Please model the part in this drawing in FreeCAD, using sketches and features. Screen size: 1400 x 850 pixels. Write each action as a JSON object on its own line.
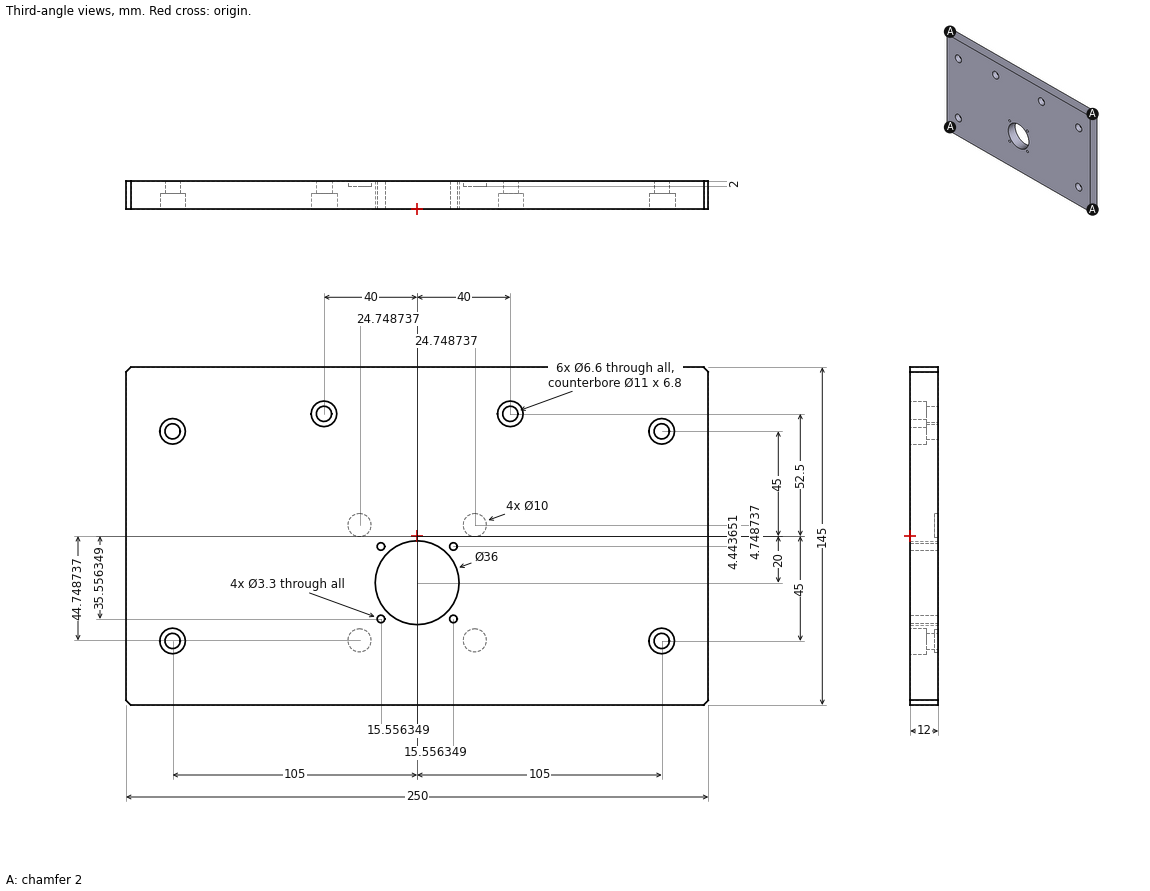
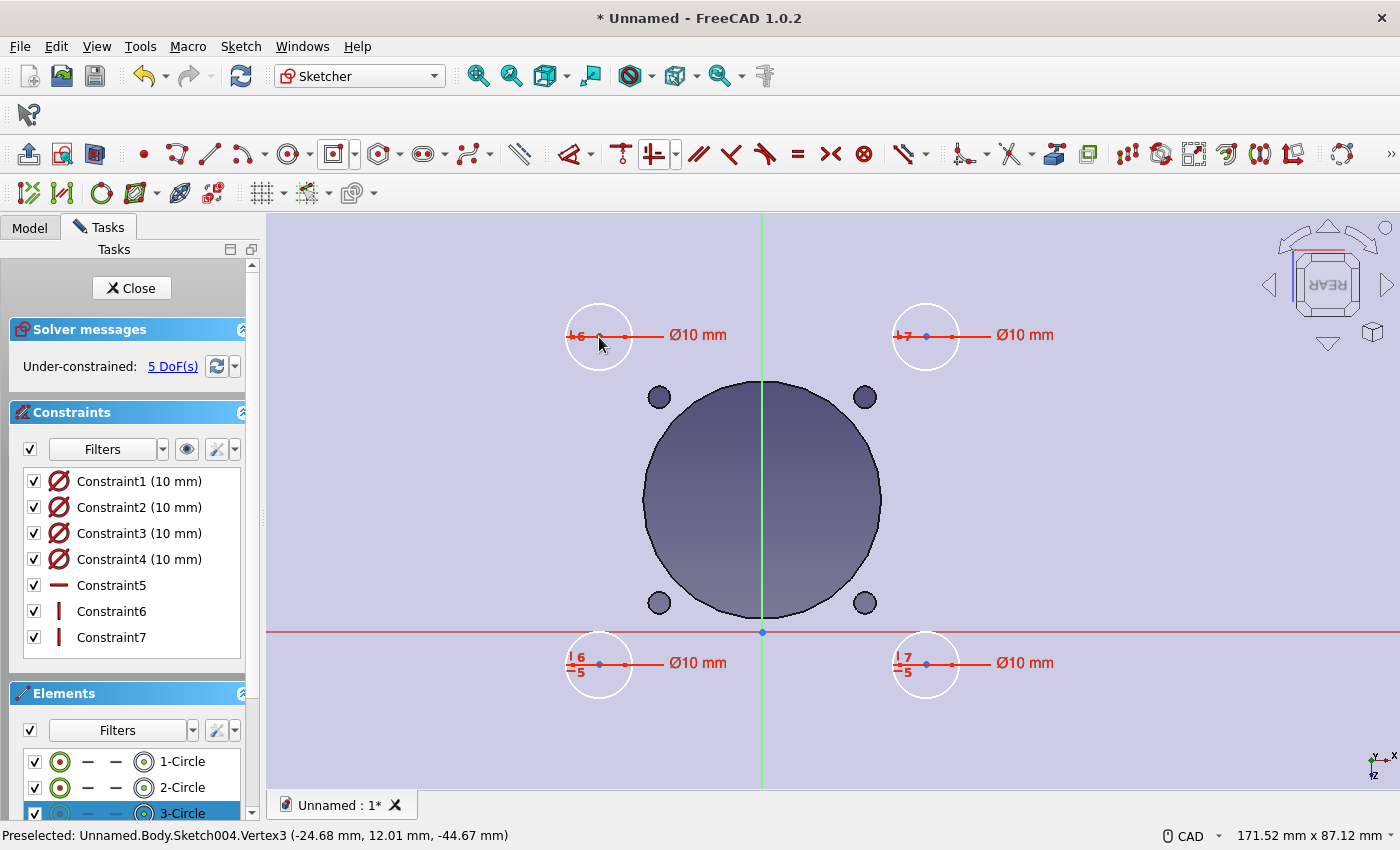
{"action": "left_click", "coordinate": [926, 337]}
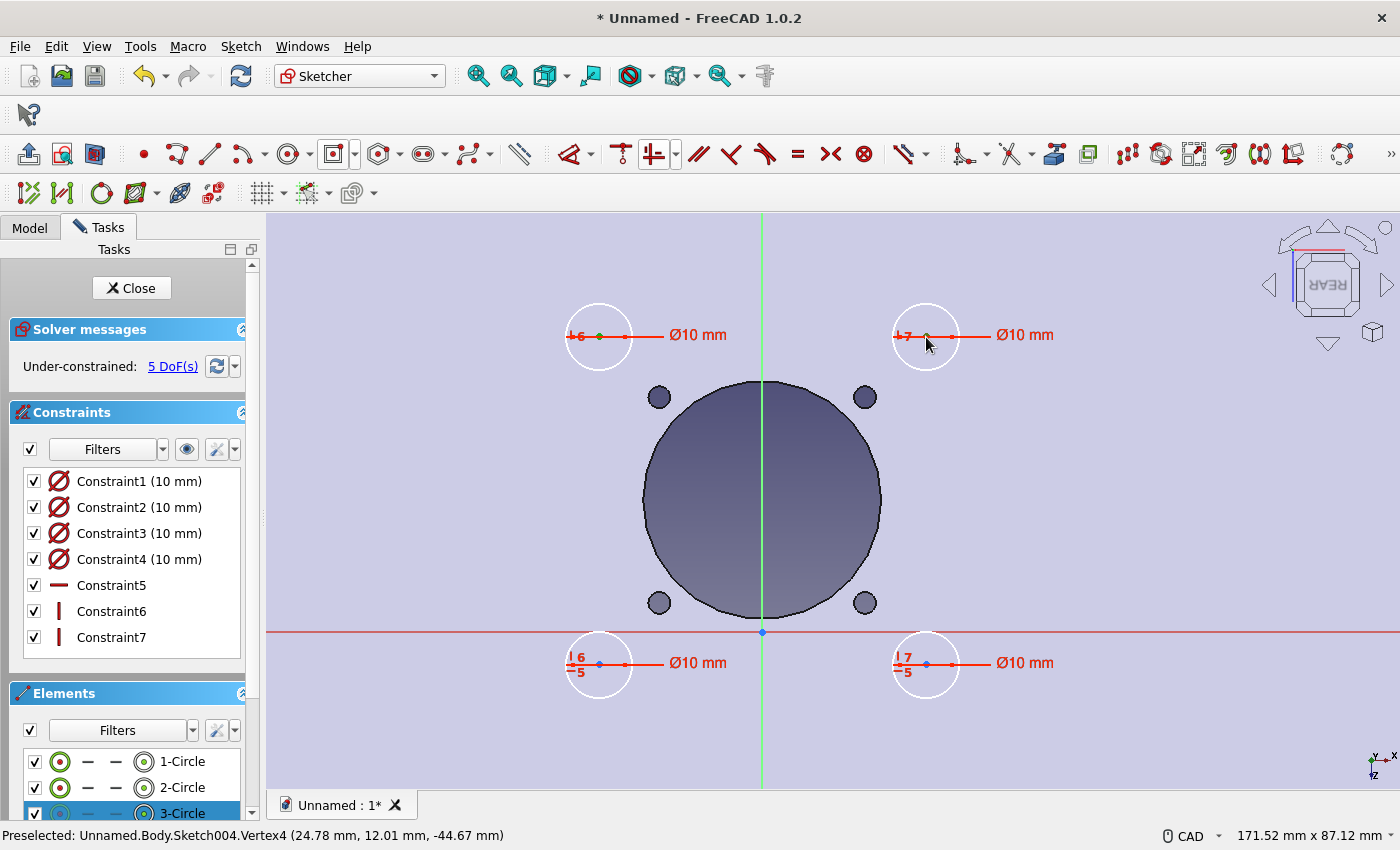
{"action": "key", "text": "h"}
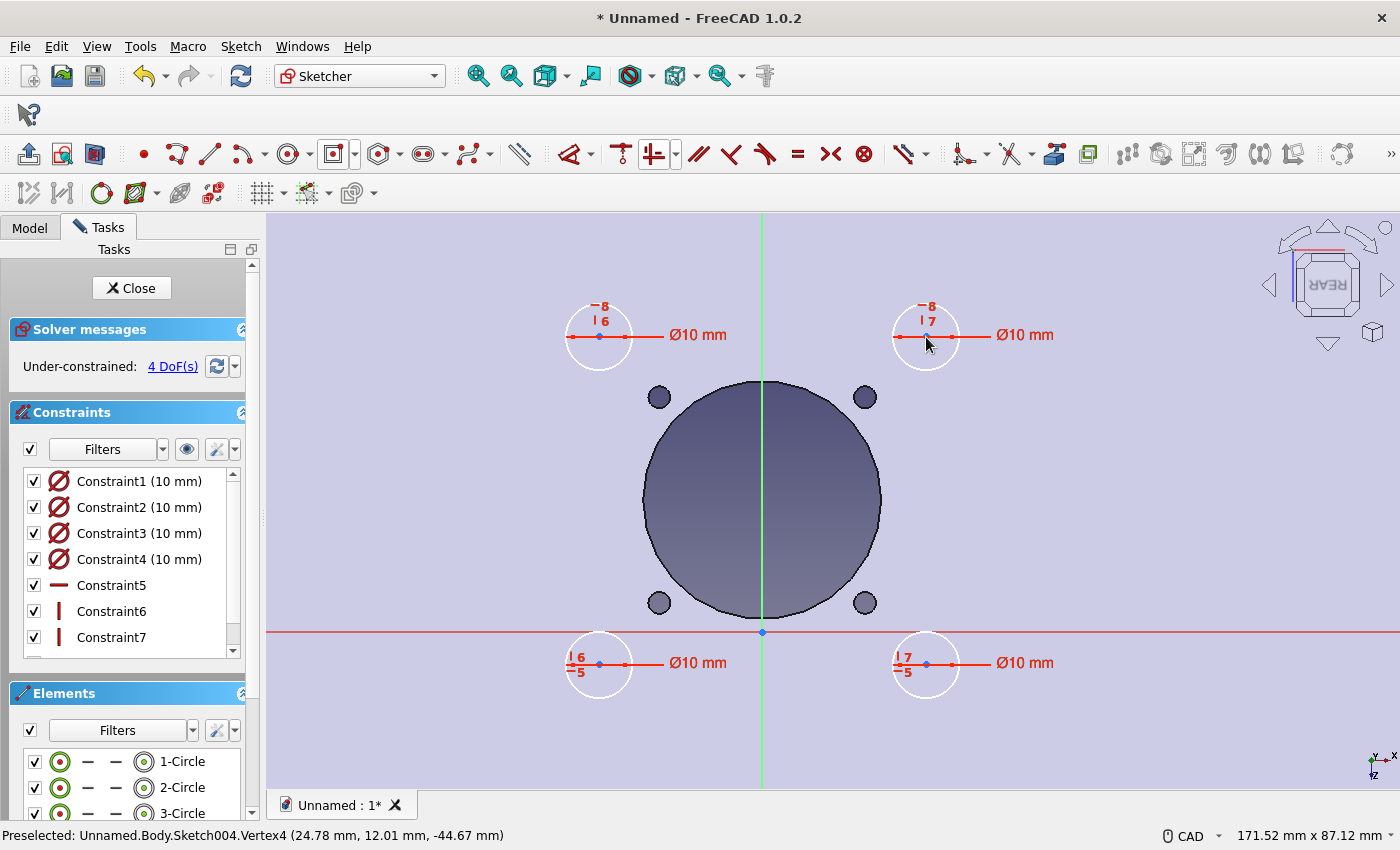
{"action": "left_click", "coordinate": [568, 154]}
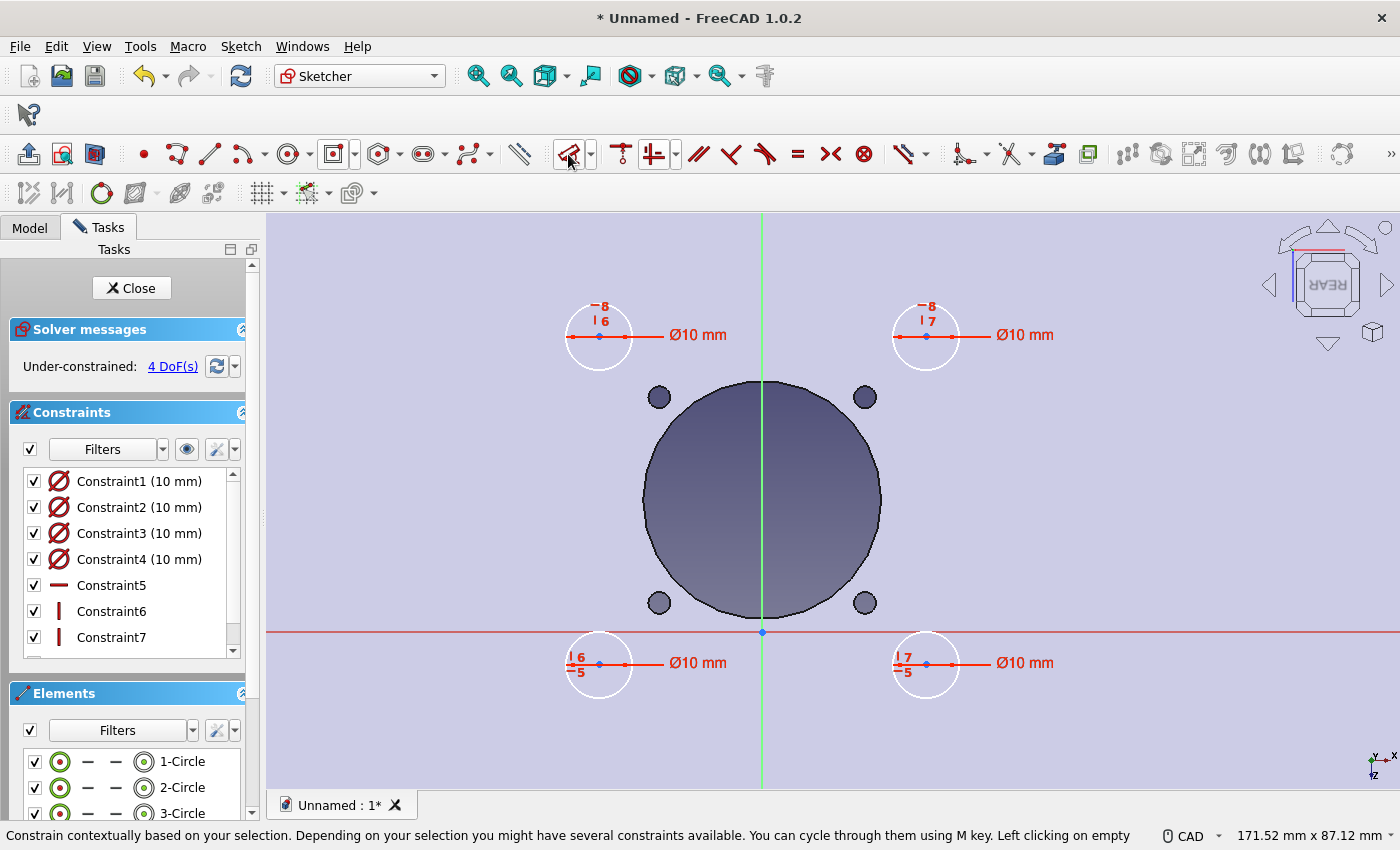
{"action": "scroll", "coordinate": [926, 665], "scroll_direction": "up", "scroll_amount": 2}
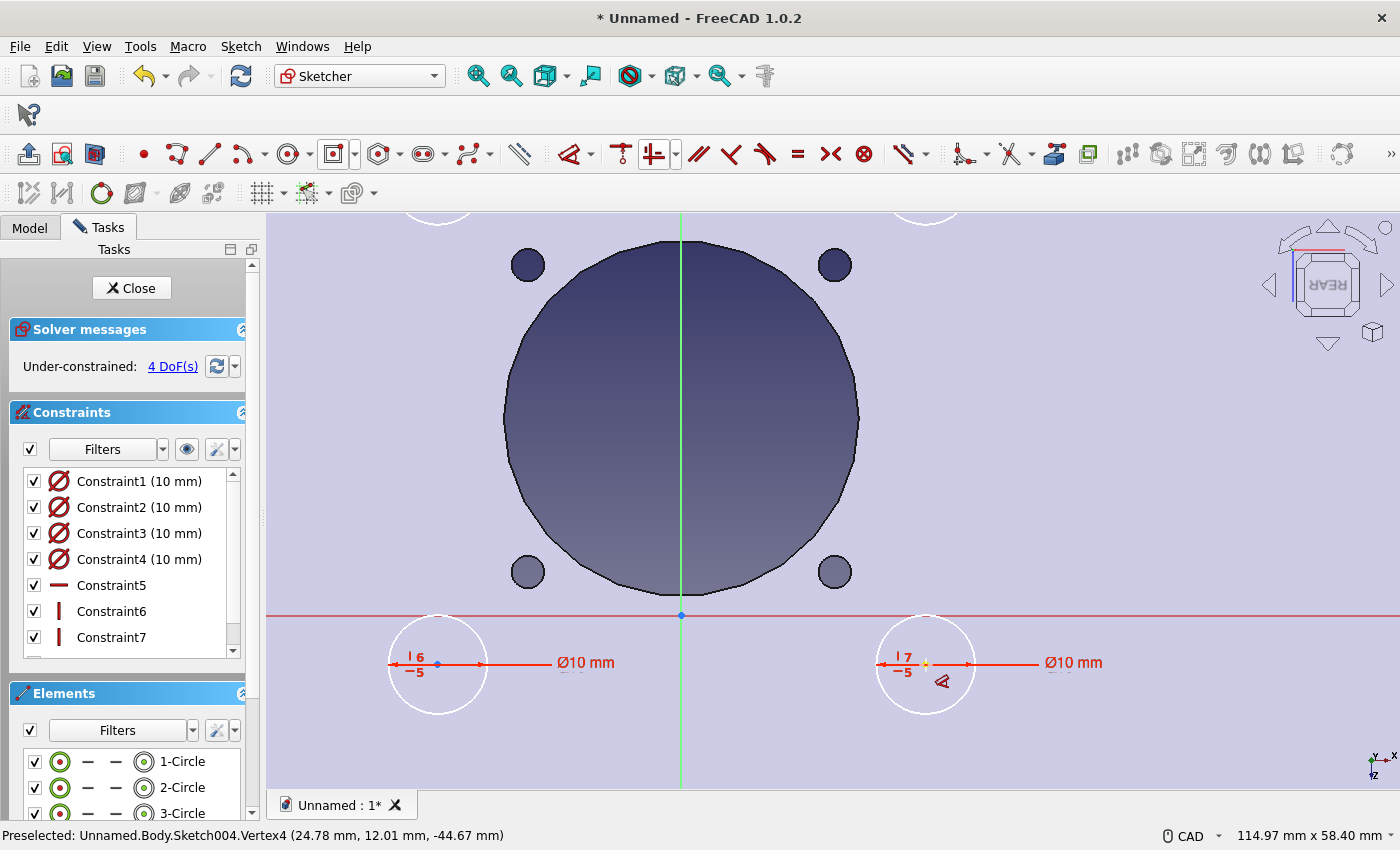
{"action": "left_click", "coordinate": [926, 665]}
{"action": "left_click", "coordinate": [960, 657]}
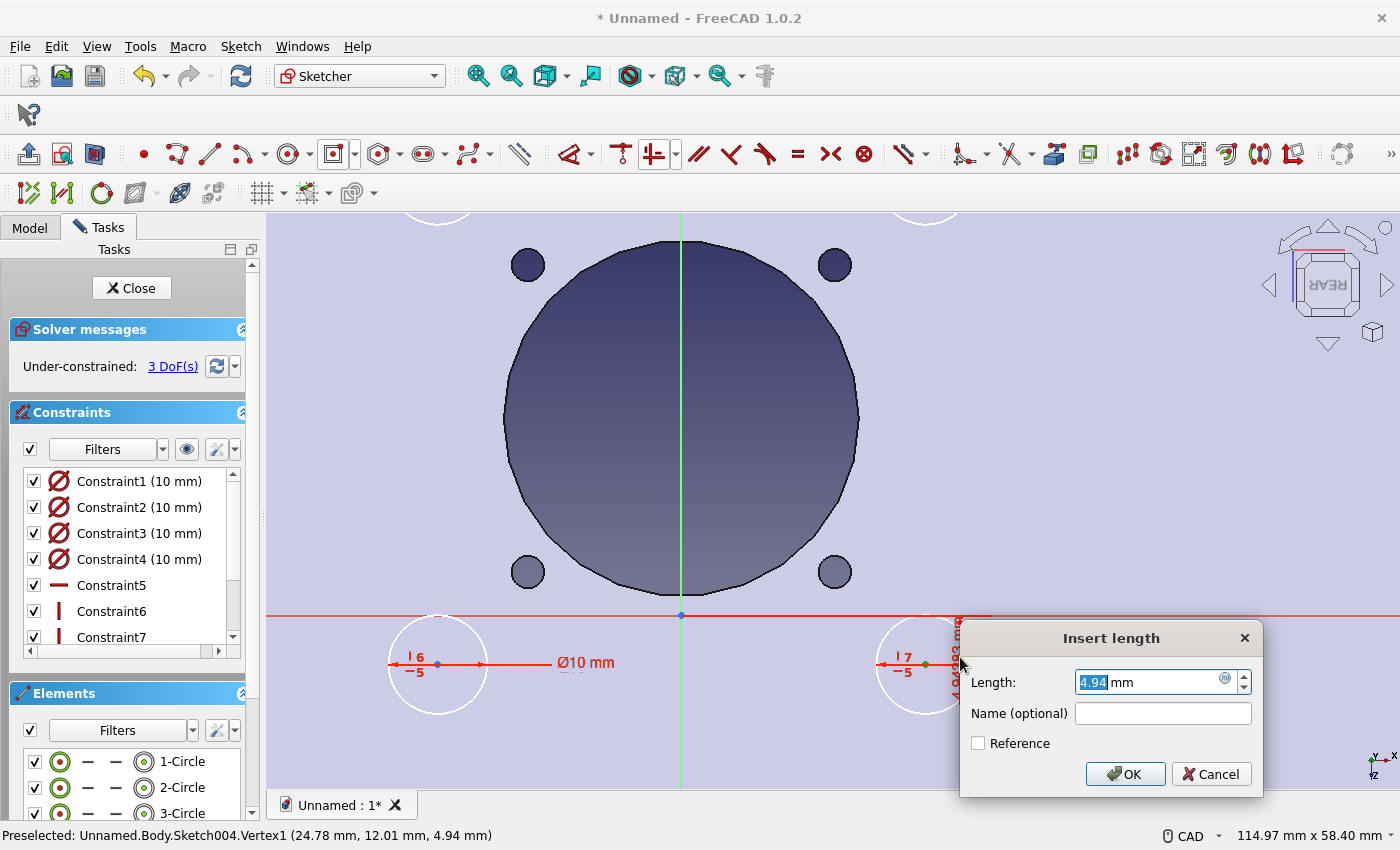
{"action": "type", "text": "4.748737"}
{"action": "key", "text": "Return"}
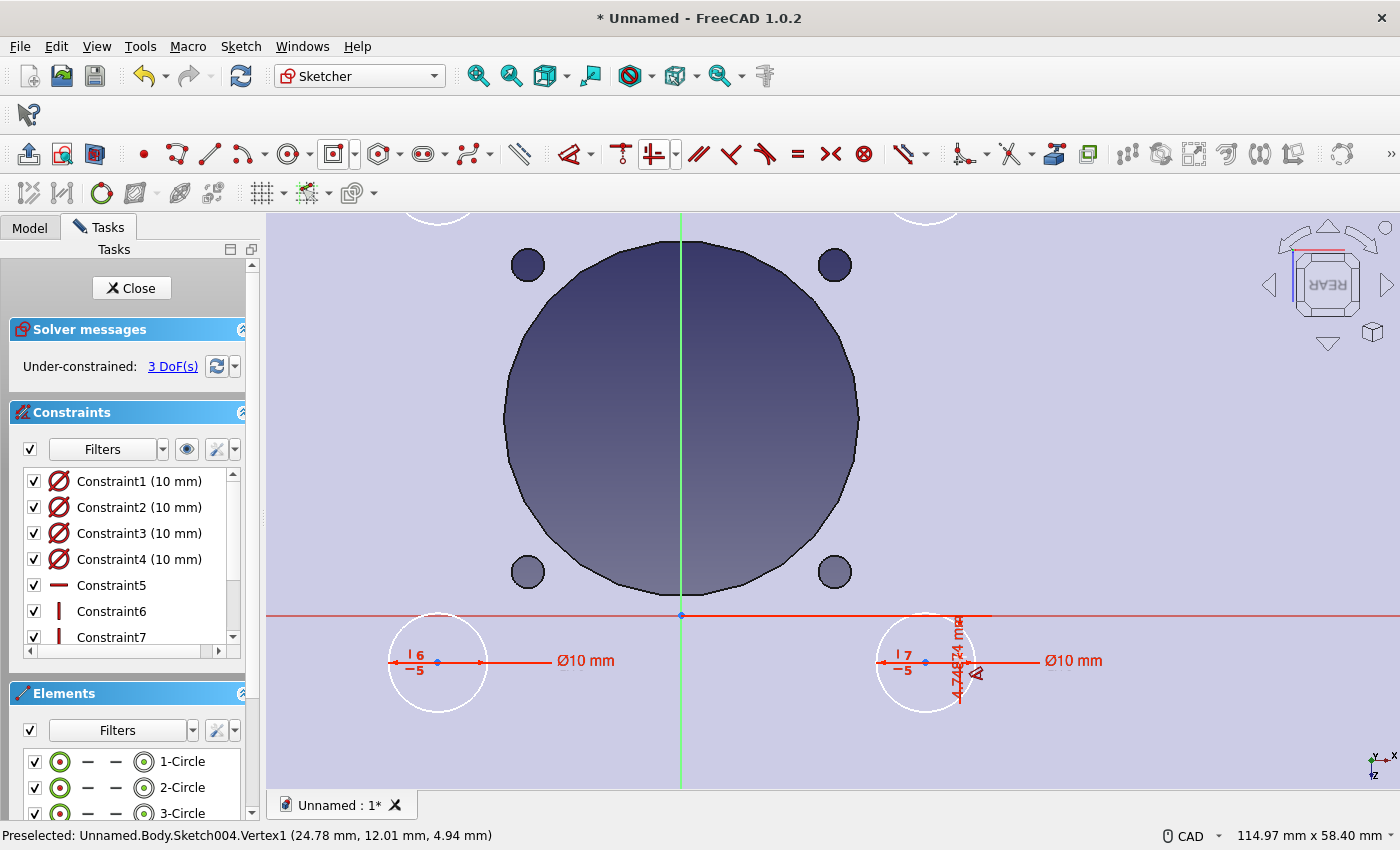
{"action": "left_click", "coordinate": [926, 663]}
{"action": "left_click", "coordinate": [804, 697]}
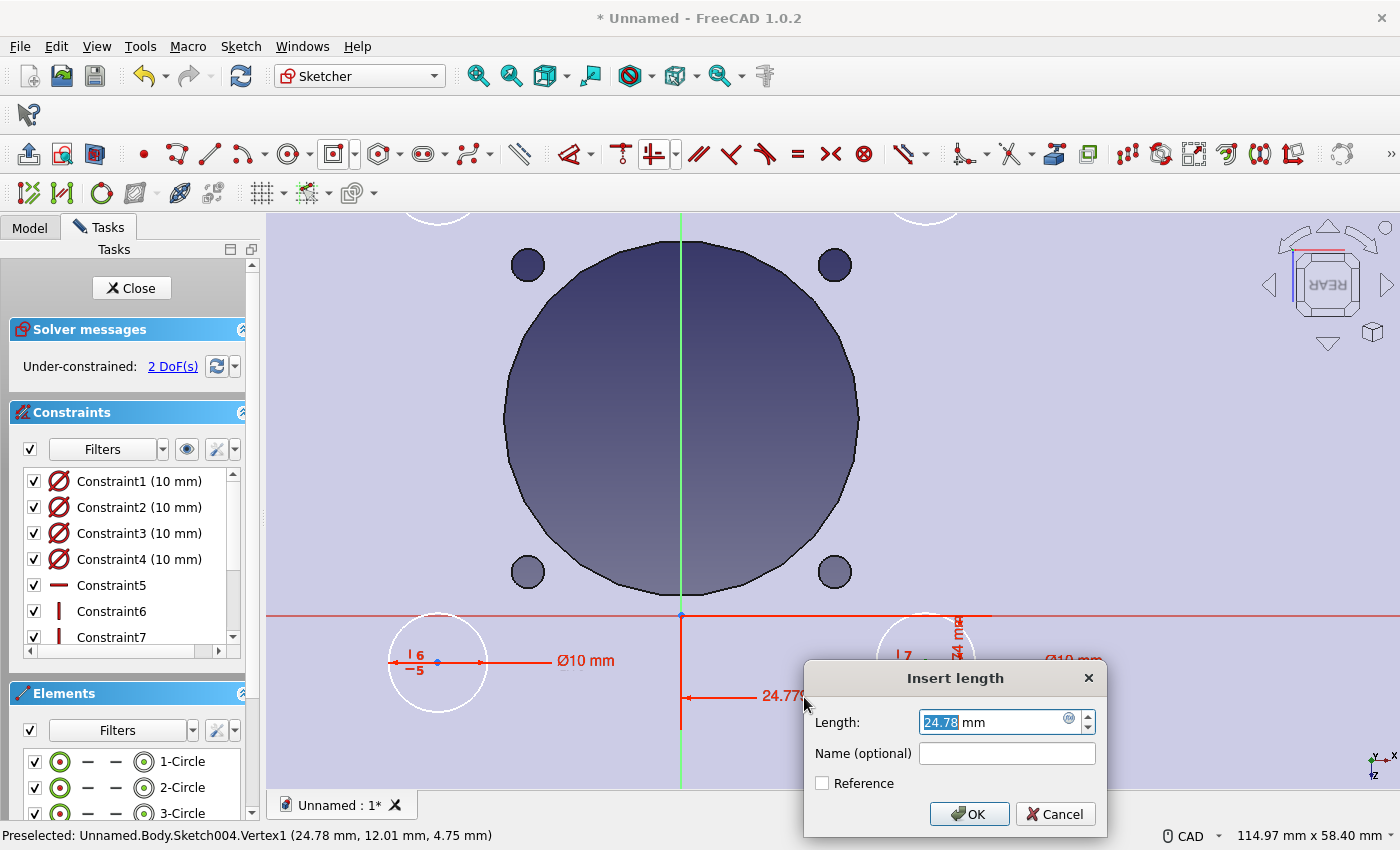
{"action": "type", "text": "24.748737"}
{"action": "key", "text": "Return"}